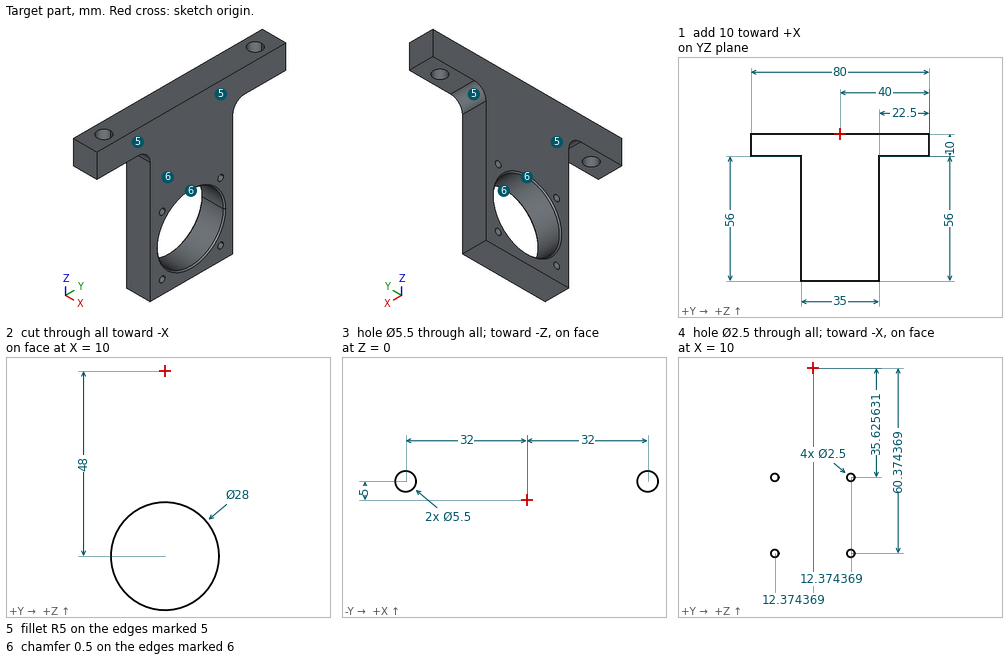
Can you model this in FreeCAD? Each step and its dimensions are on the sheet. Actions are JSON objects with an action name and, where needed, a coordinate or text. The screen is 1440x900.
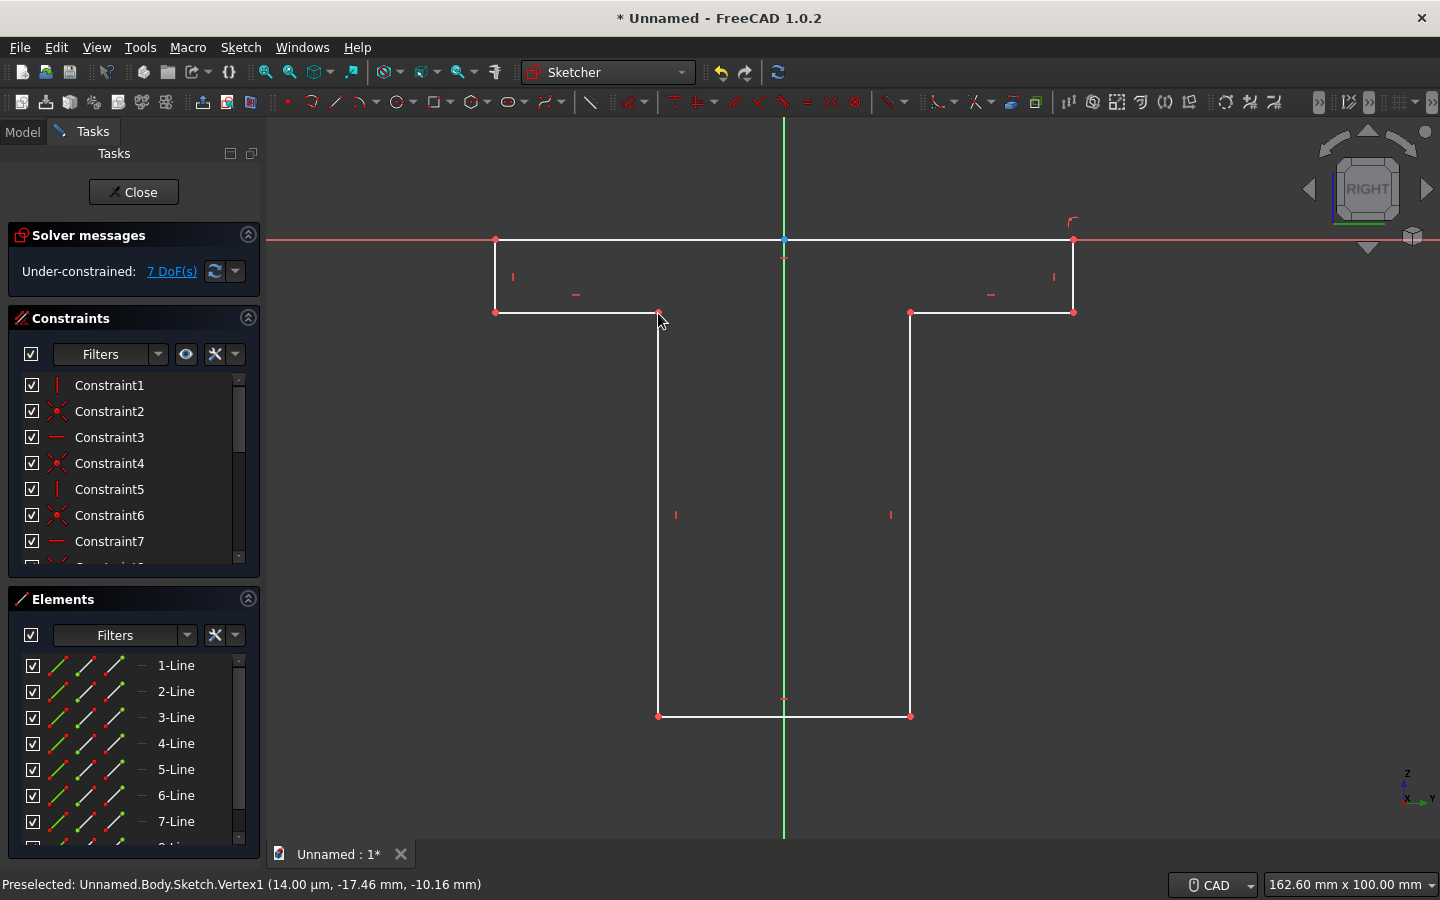
{"action": "left_click", "coordinate": [628, 102]}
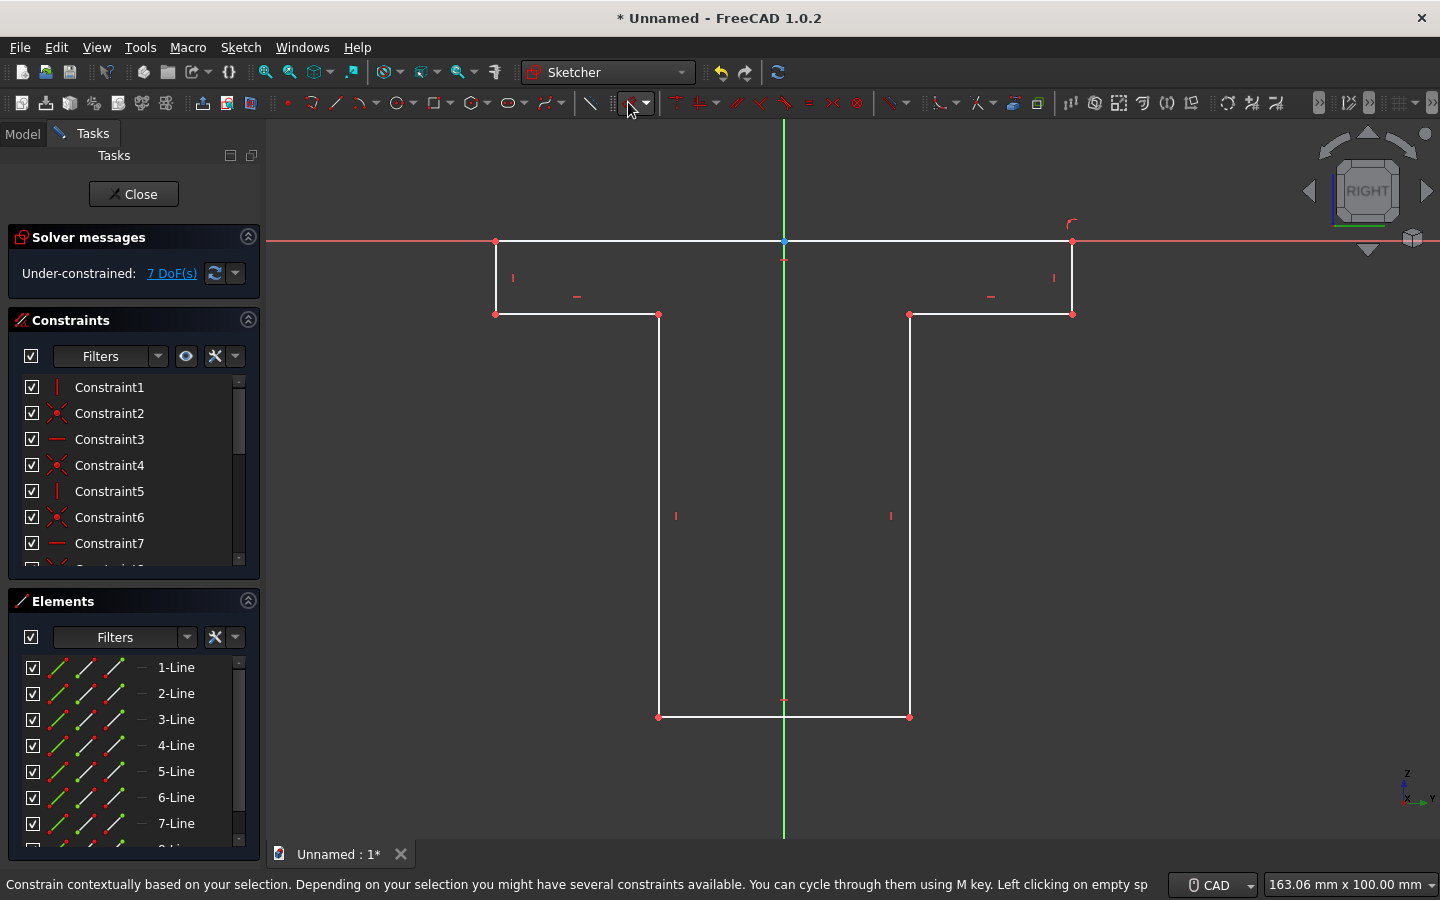
{"action": "left_click", "coordinate": [659, 435]}
{"action": "left_click", "coordinate": [625, 516]}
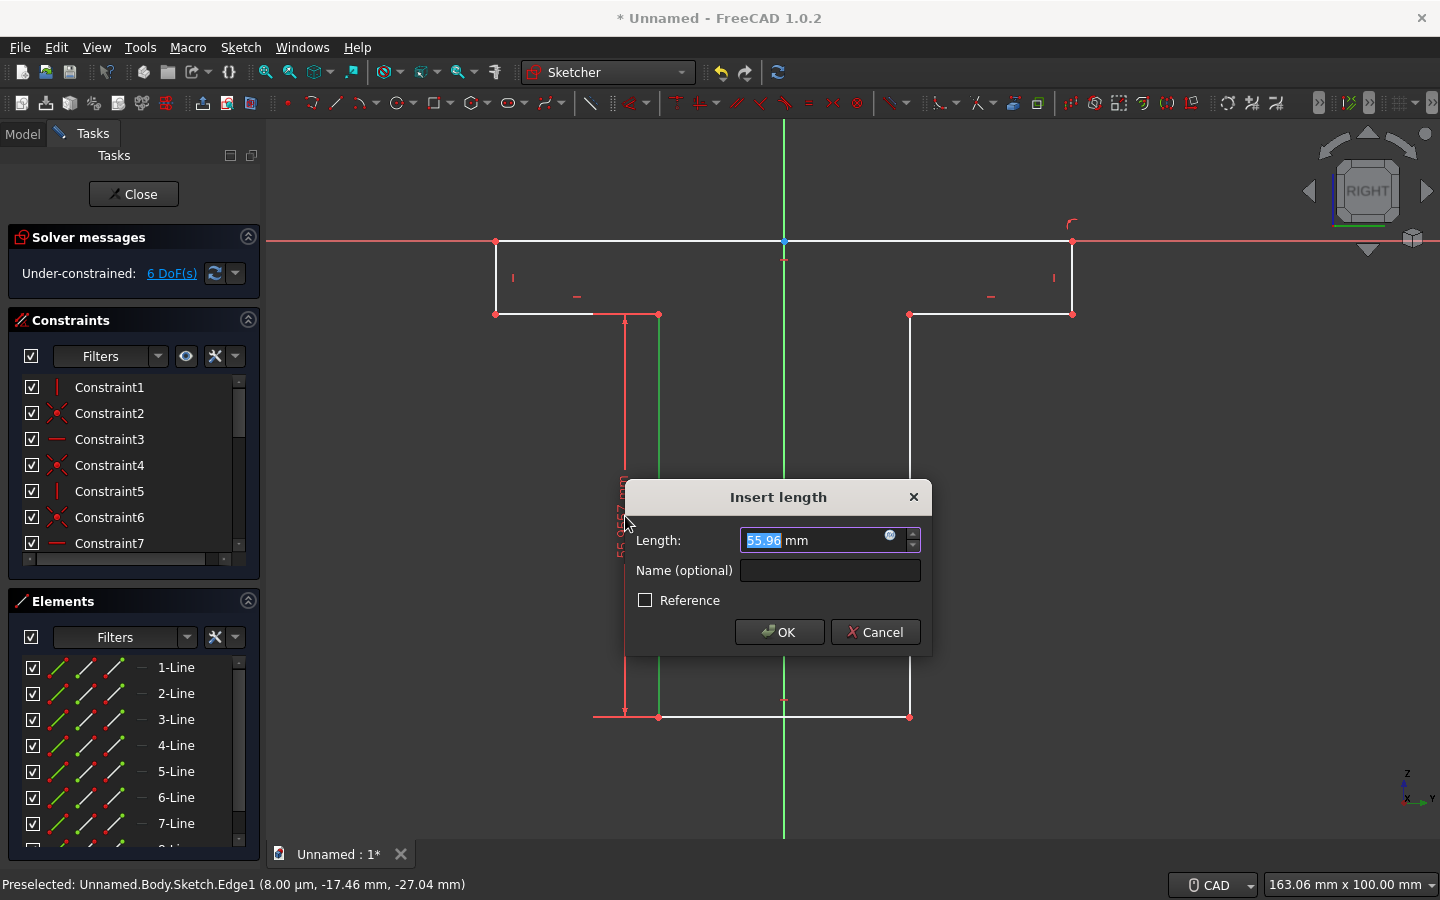
{"action": "type", "text": "56"}
{"action": "key", "text": "Return"}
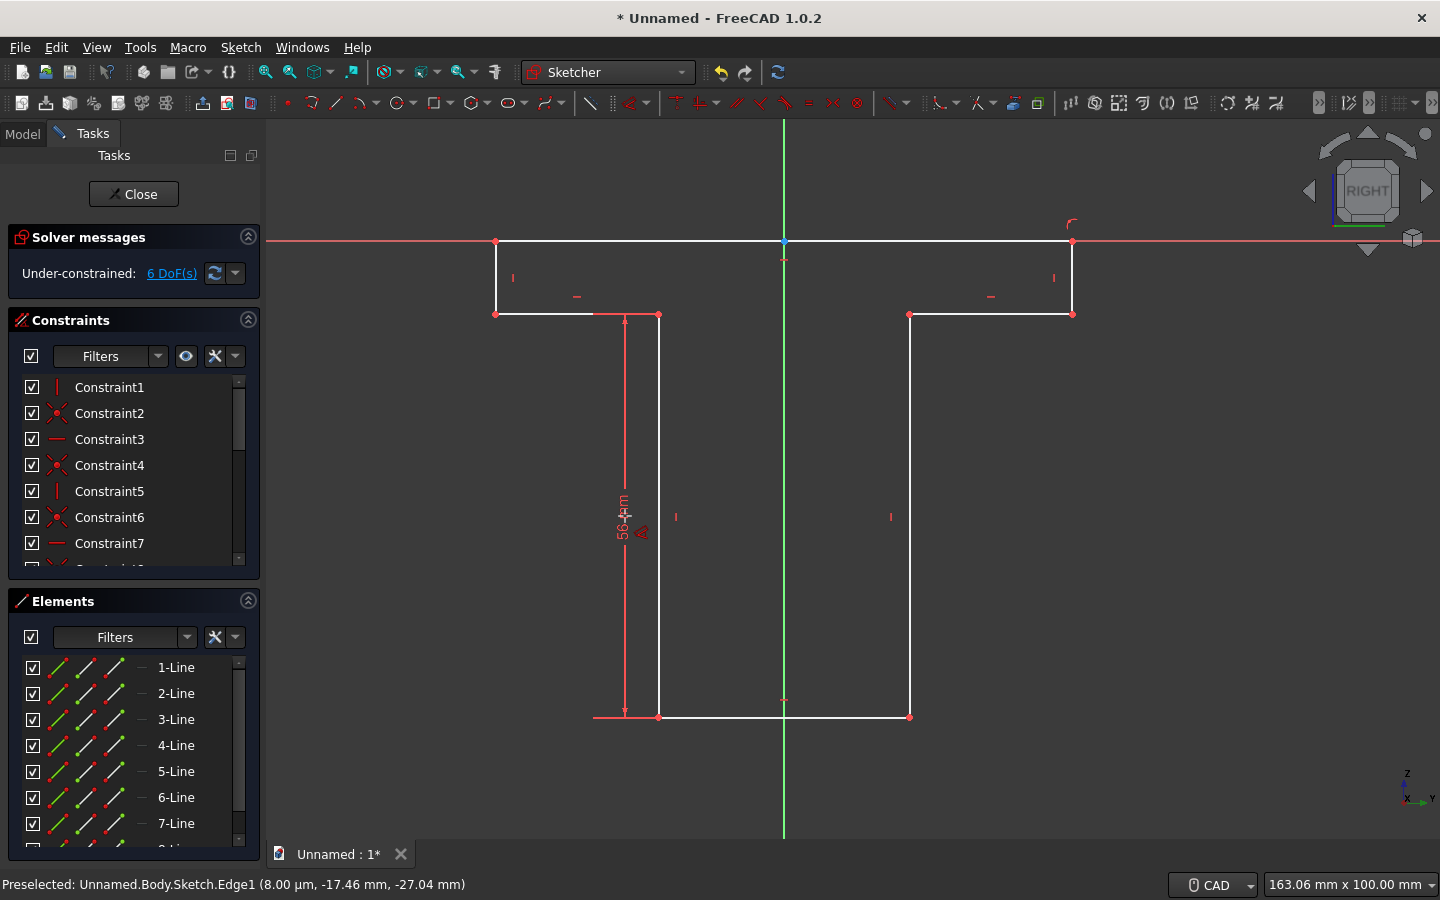
{"action": "left_click", "coordinate": [734, 718]}
{"action": "left_click", "coordinate": [726, 752]}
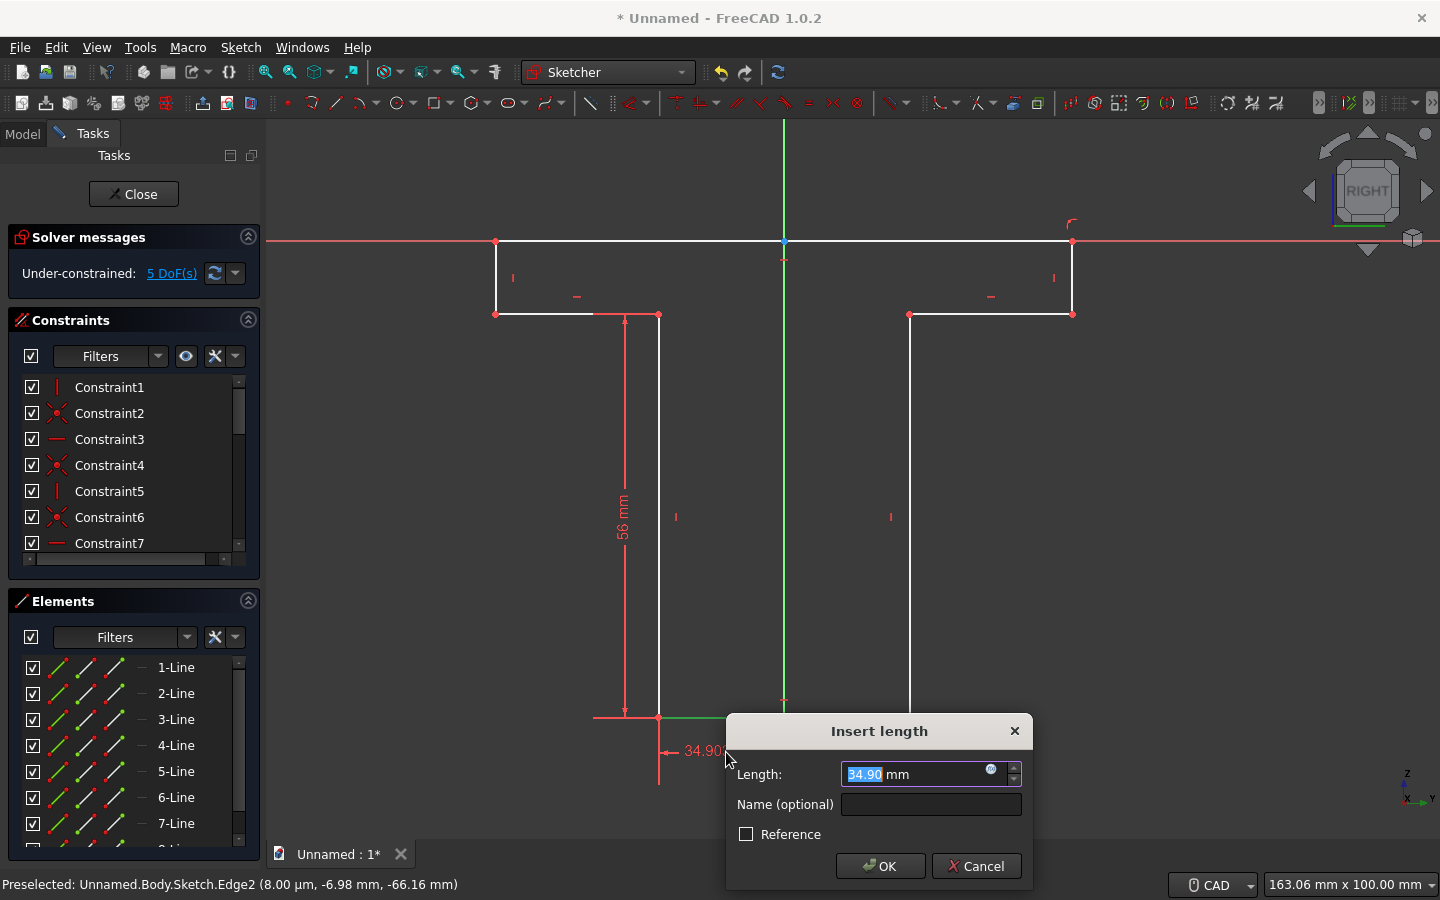
{"action": "type", "text": "35"}
{"action": "key", "text": "Return"}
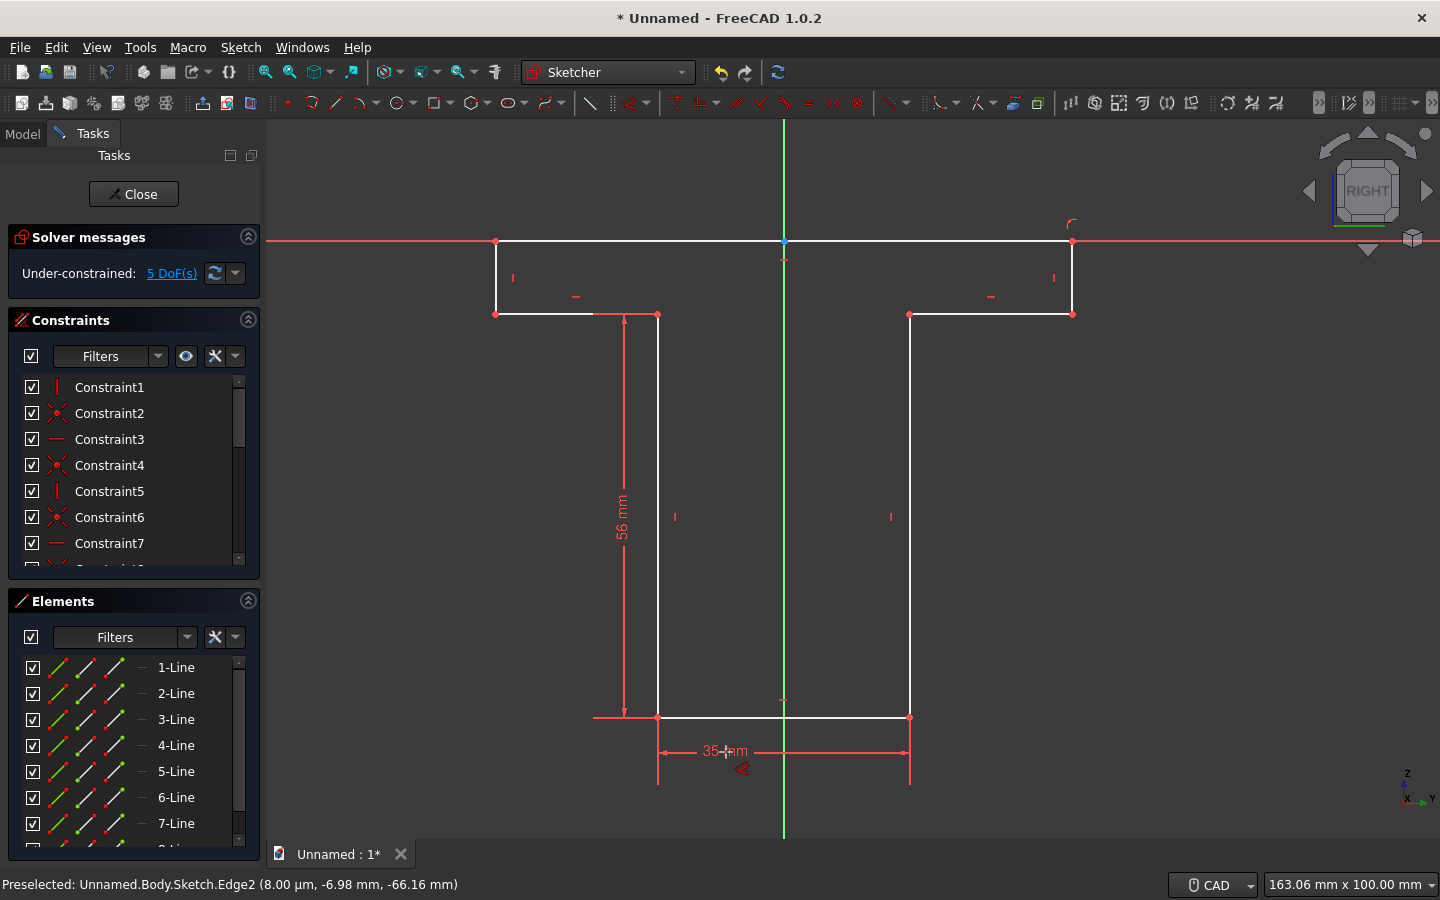
{"action": "left_click", "coordinate": [910, 597]}
{"action": "left_click", "coordinate": [944, 516]}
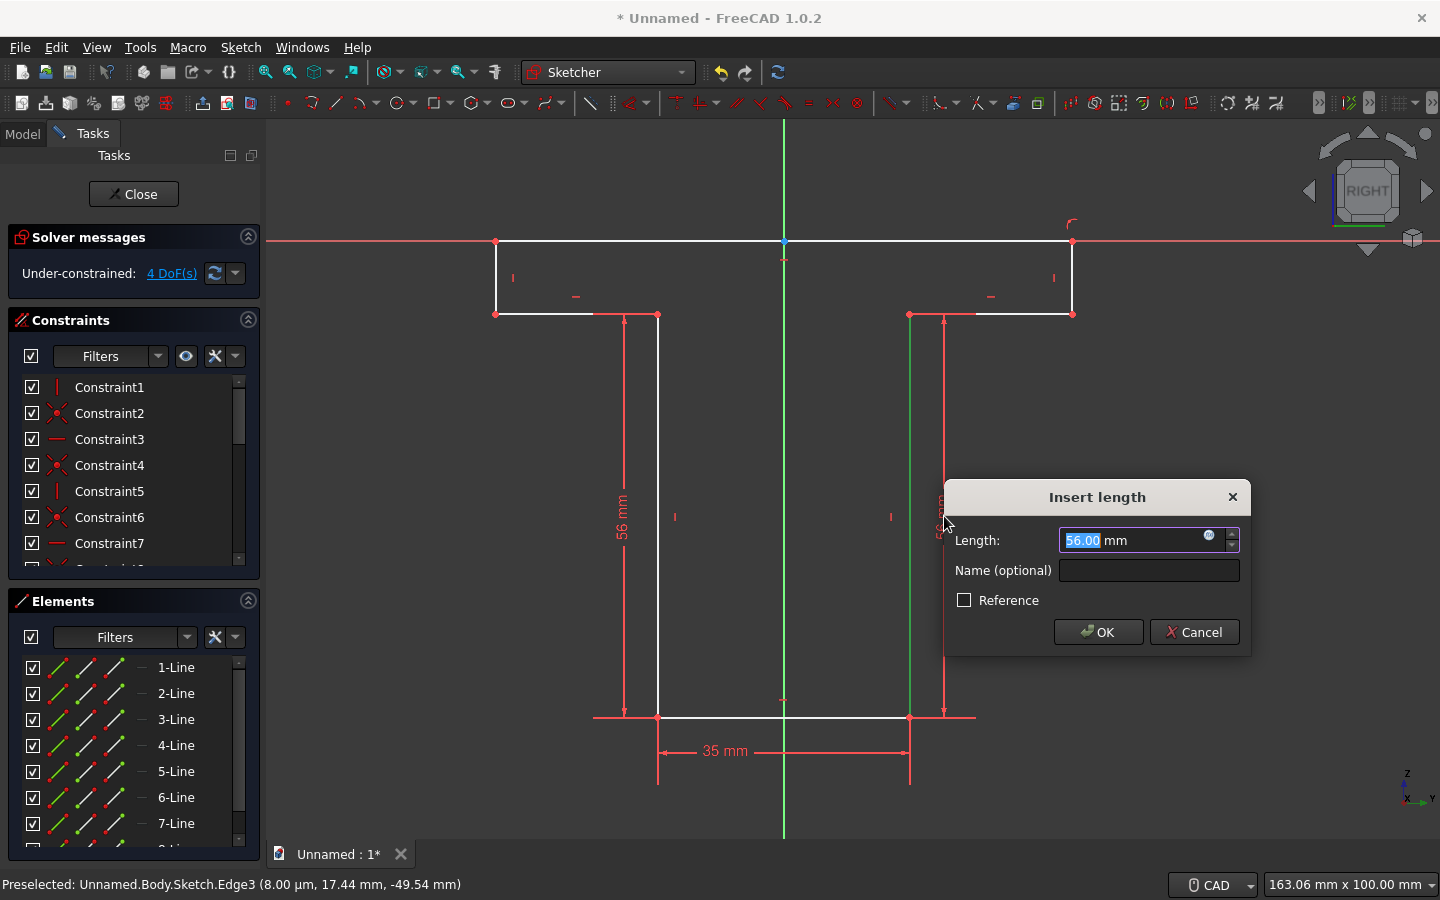
{"action": "type", "text": "56"}
{"action": "key", "text": "Return"}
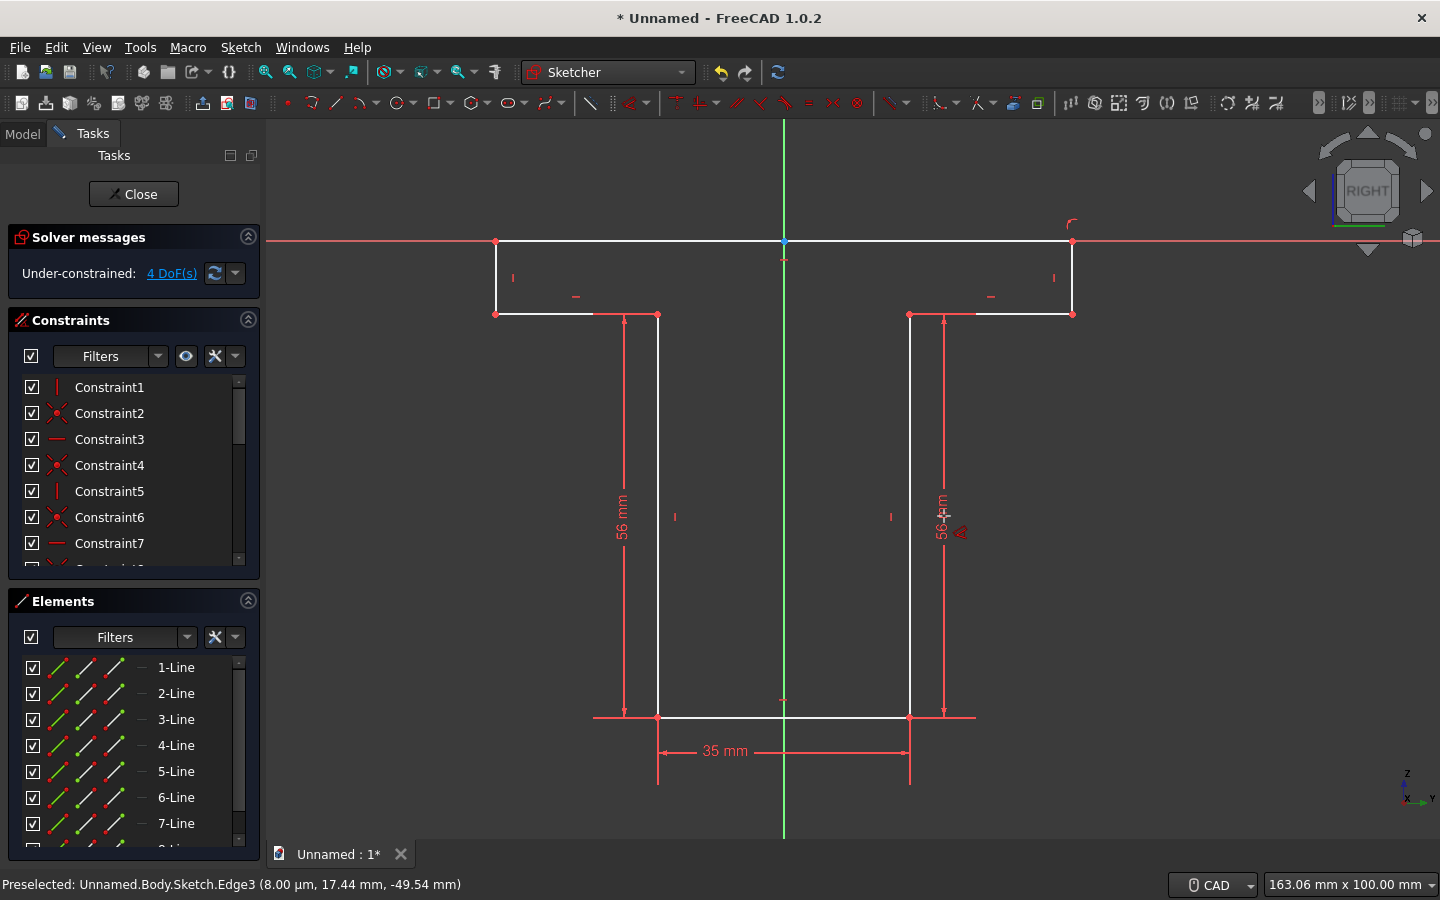
{"action": "left_click", "coordinate": [1072, 293]}
{"action": "left_click", "coordinate": [1106, 278]}